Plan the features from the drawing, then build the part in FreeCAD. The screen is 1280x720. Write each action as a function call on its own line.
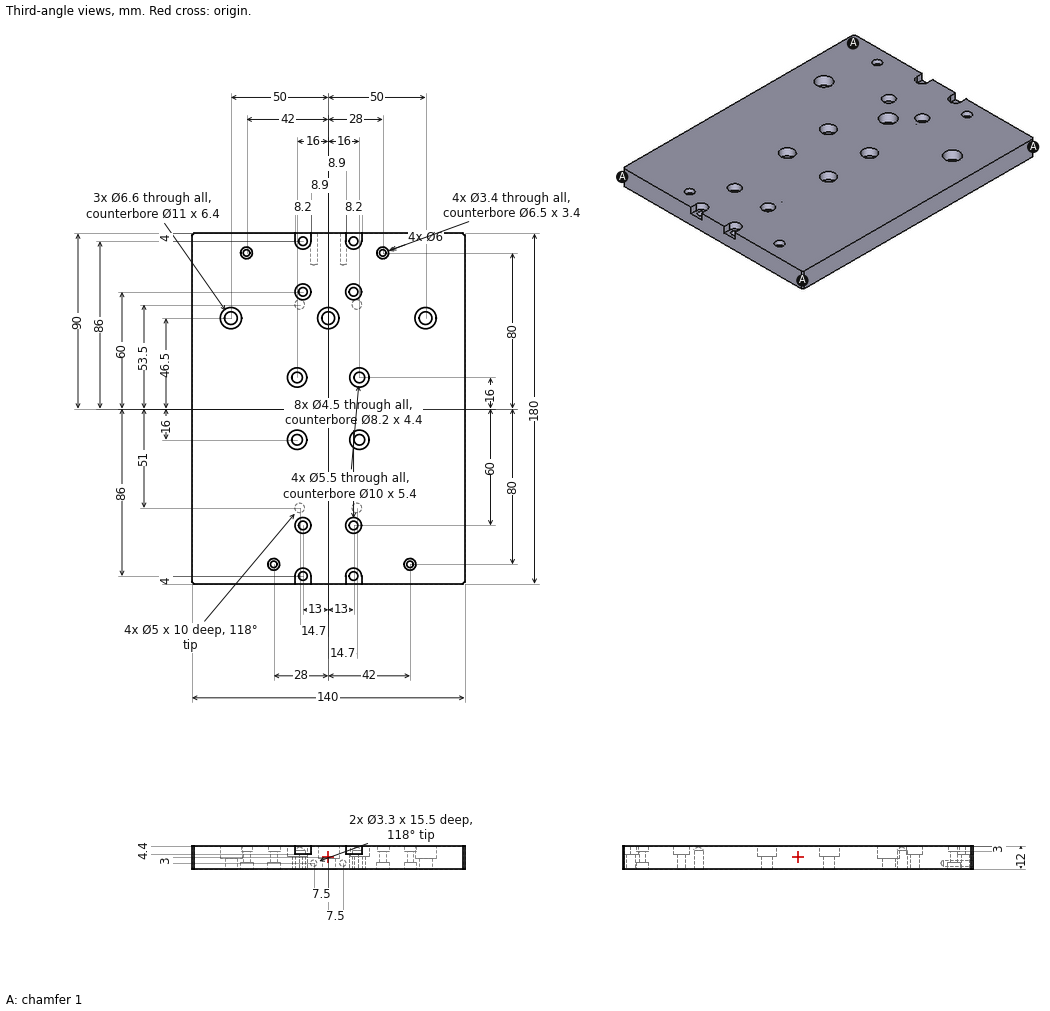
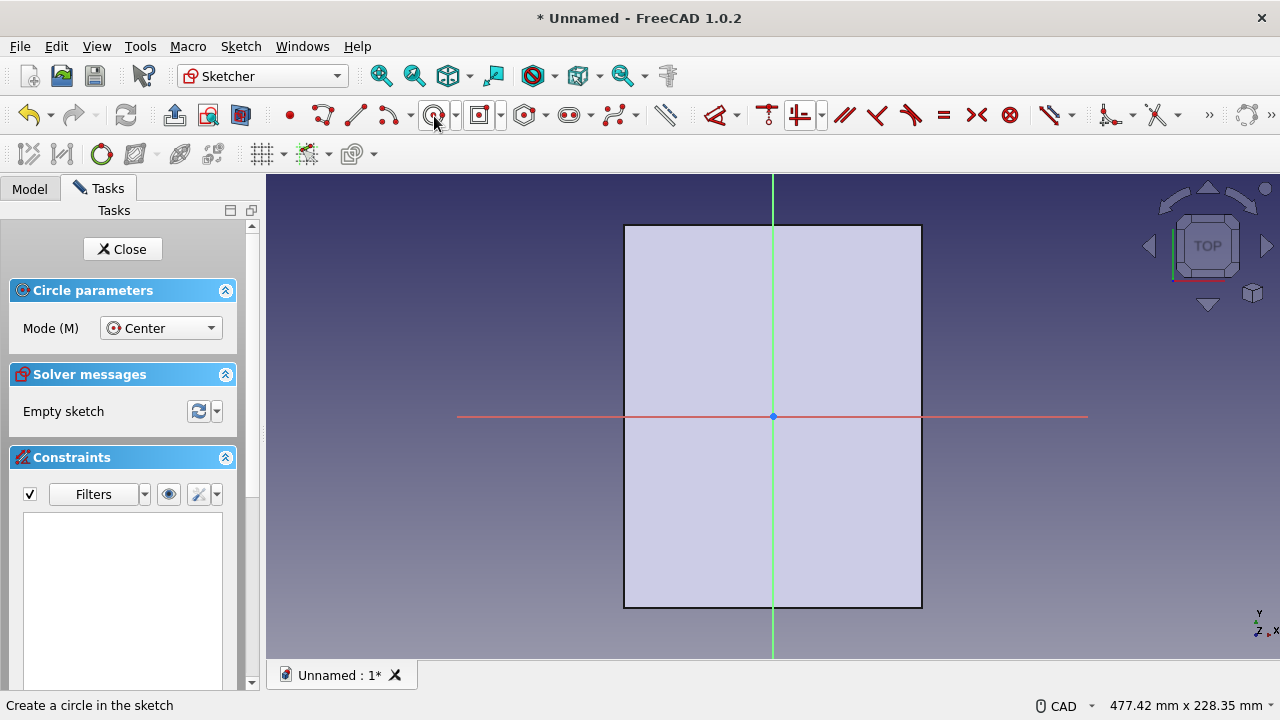
scroll(801, 544, up, 8)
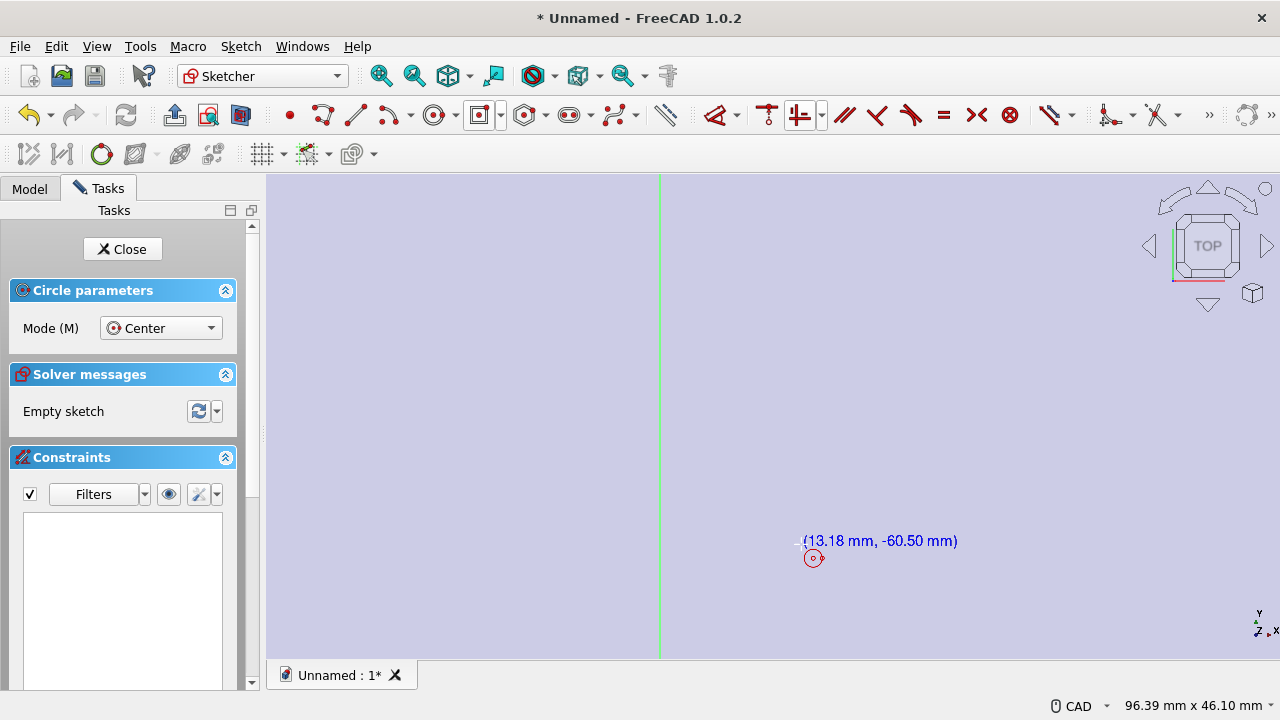
scroll(713, 517, down, 9)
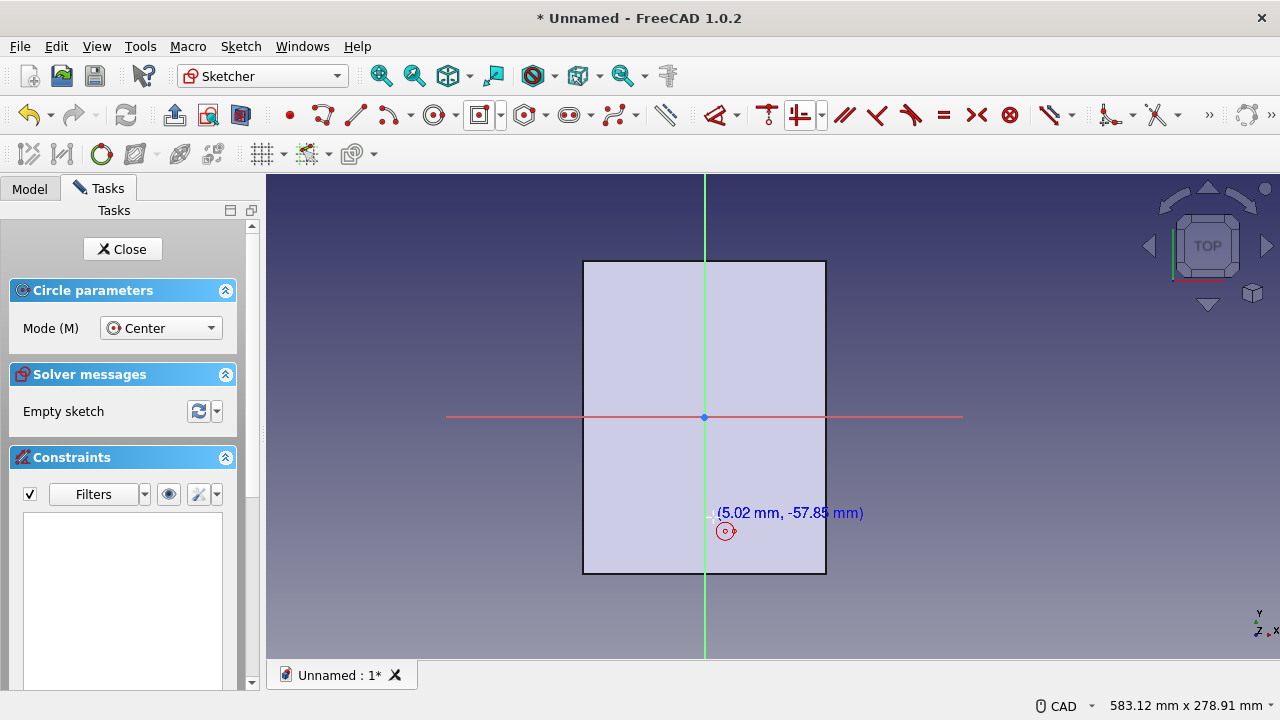
click(727, 522)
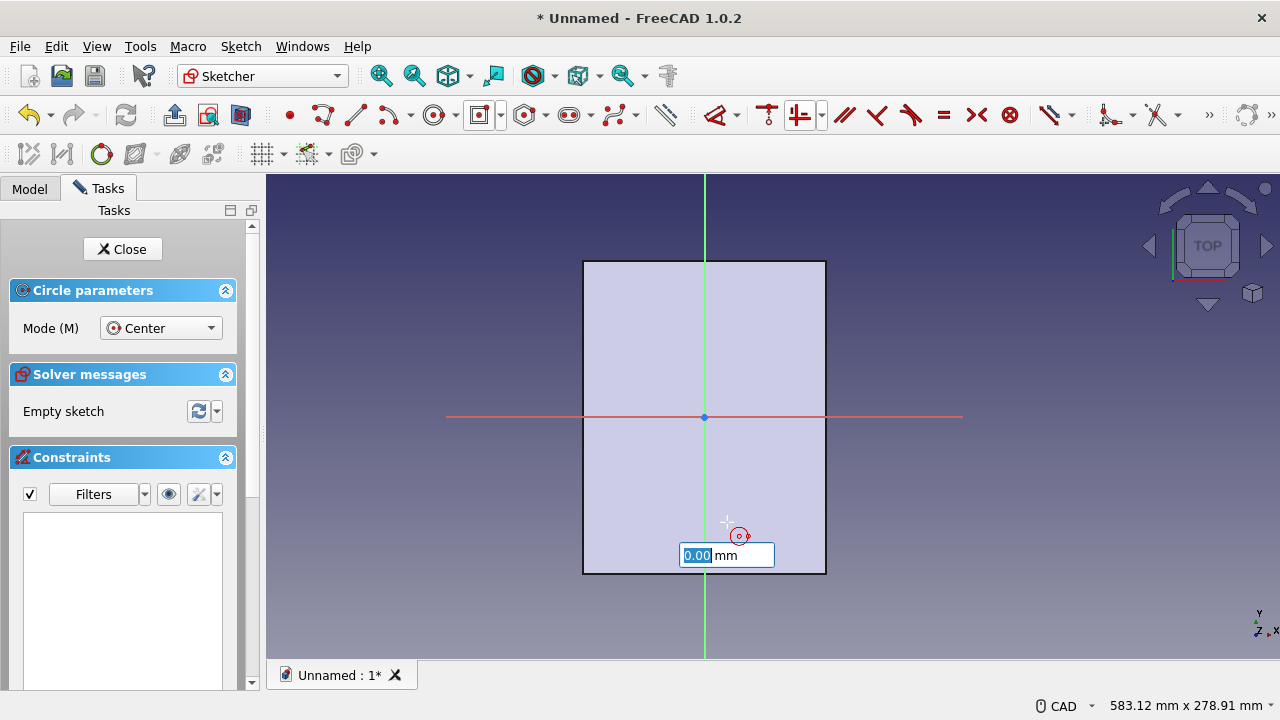
scroll(730, 519, up, 8)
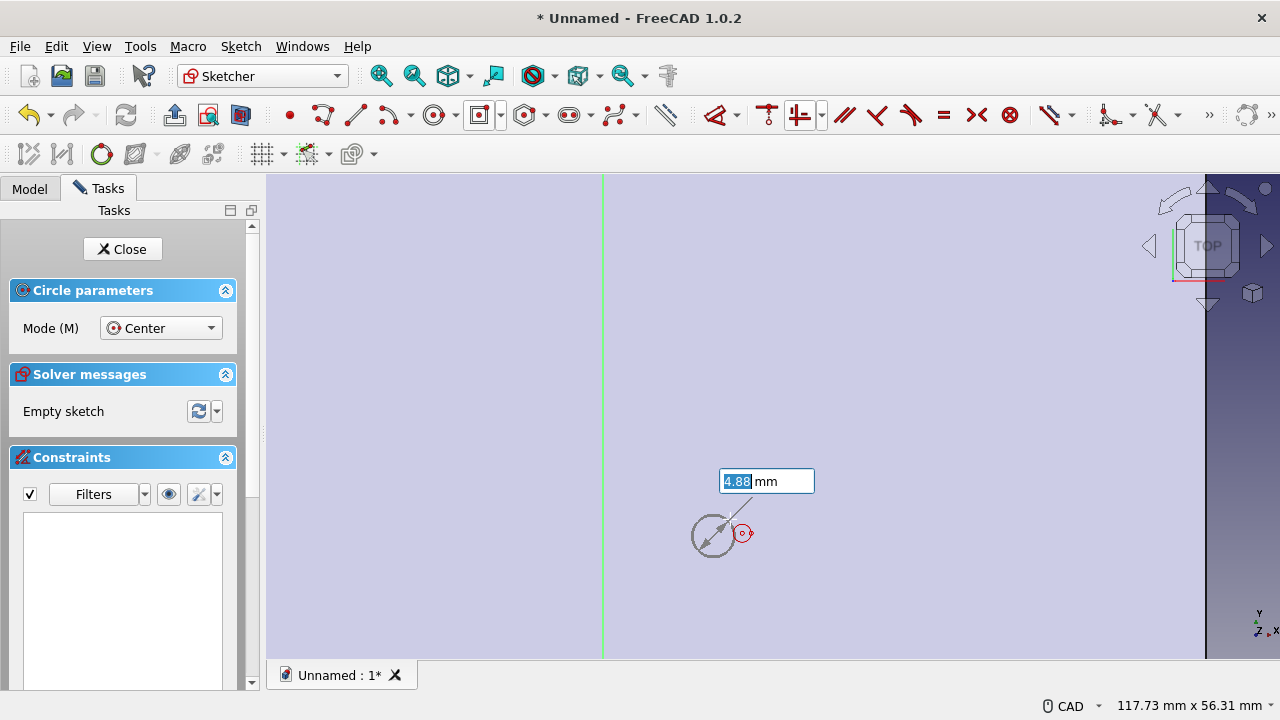
click(728, 515)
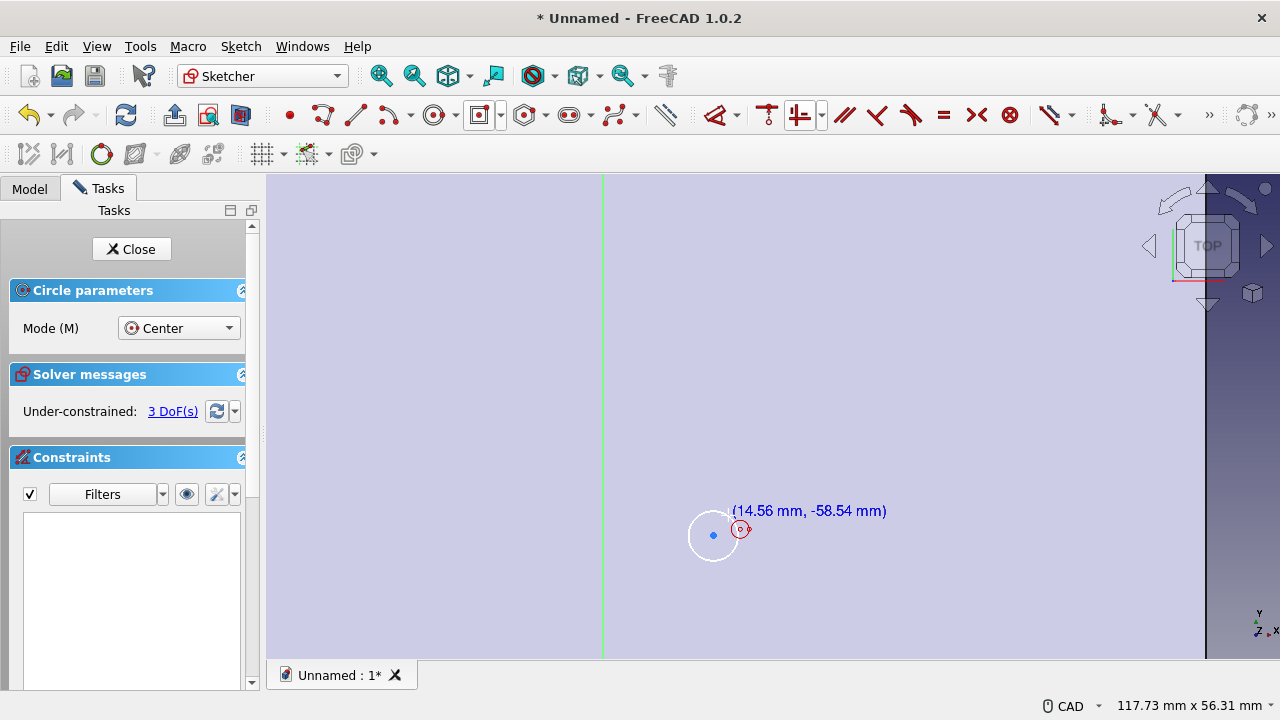
scroll(730, 519, down, 8)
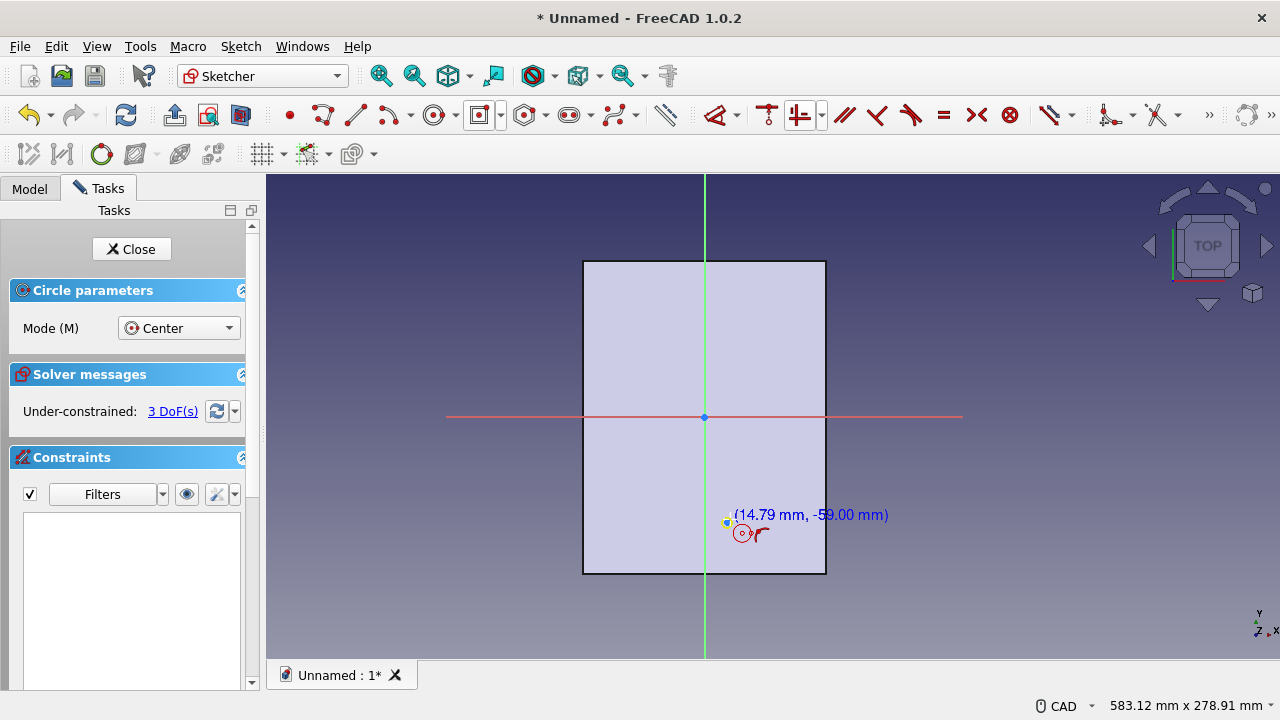
click(682, 522)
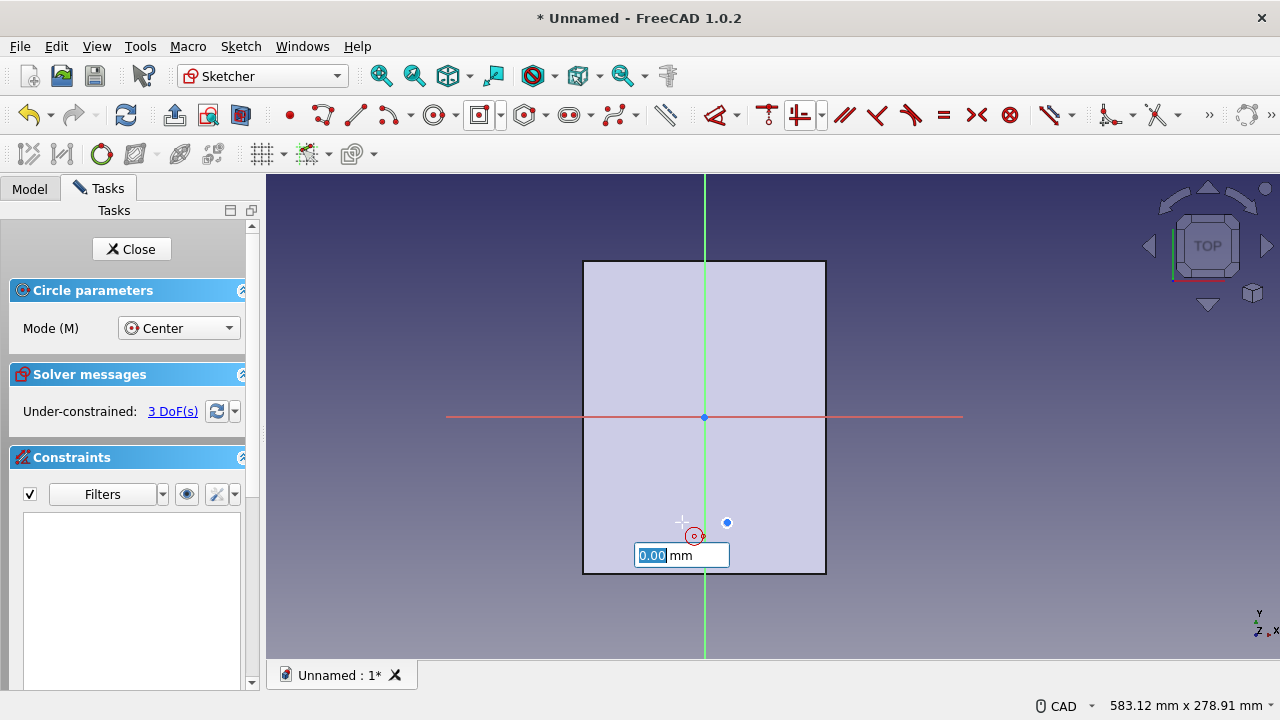
scroll(685, 519, up, 8)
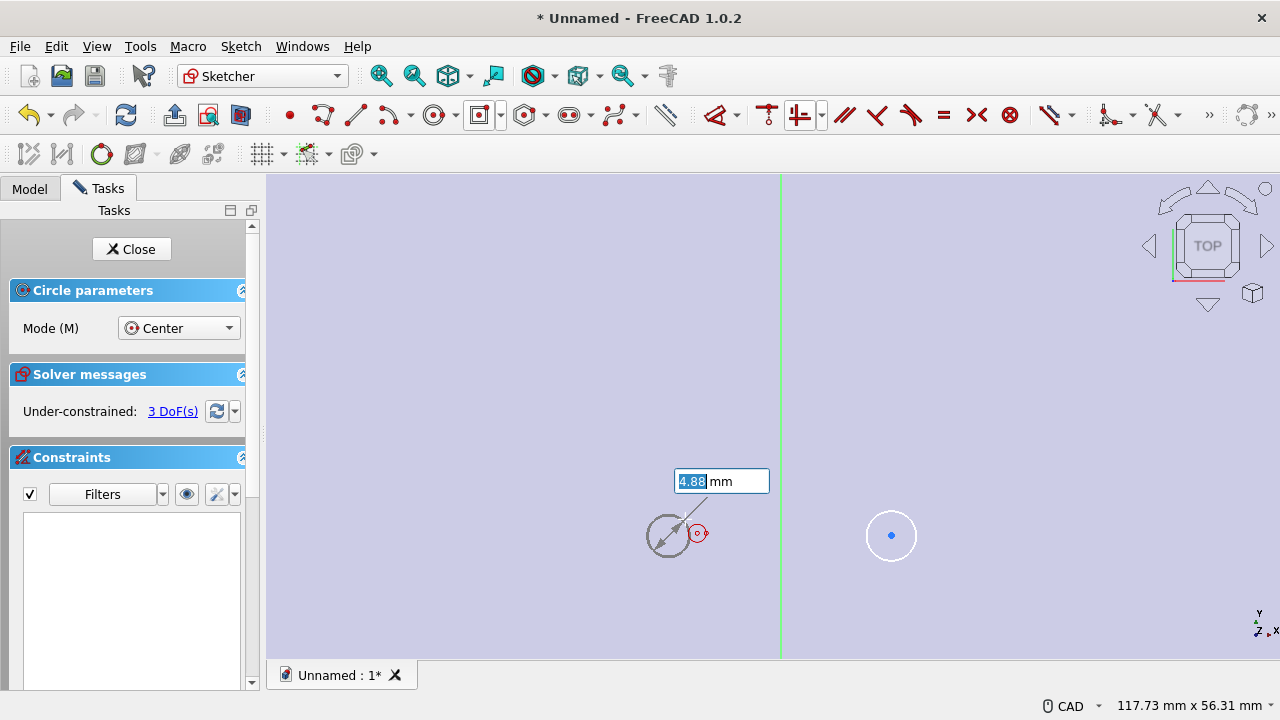
click(682, 515)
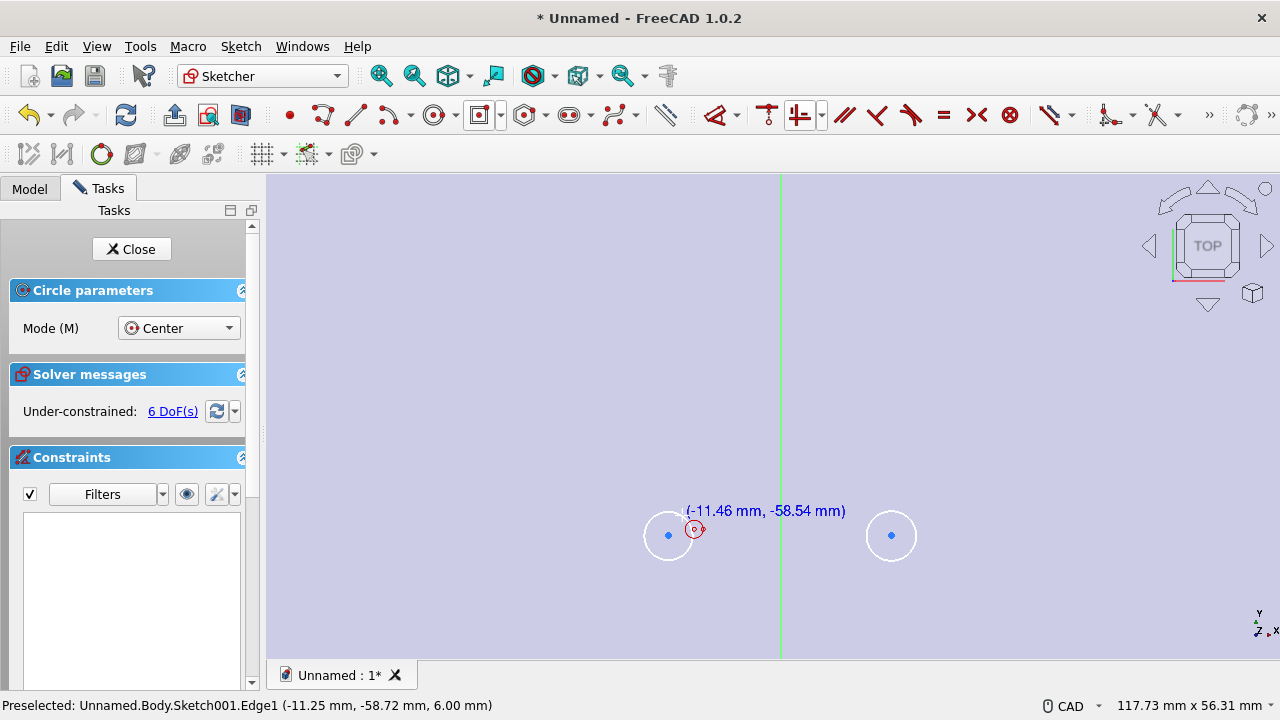
scroll(685, 519, down, 8)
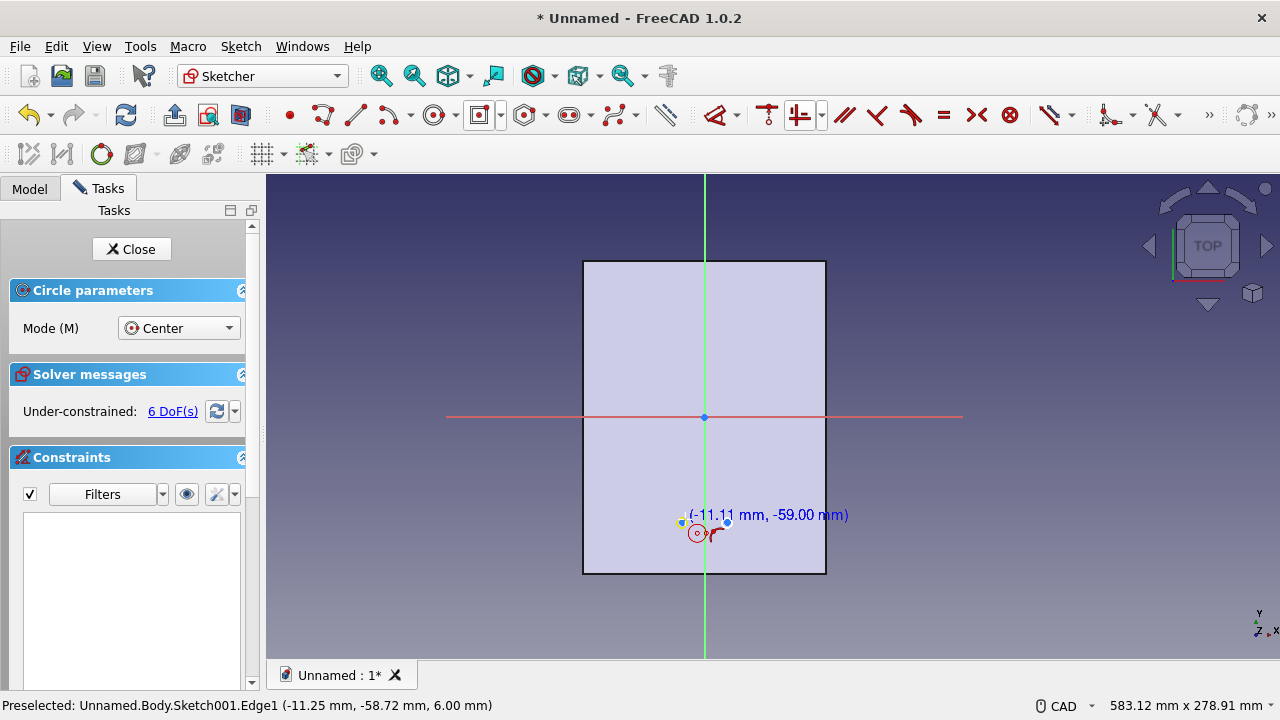
scroll(682, 567, up, 9)